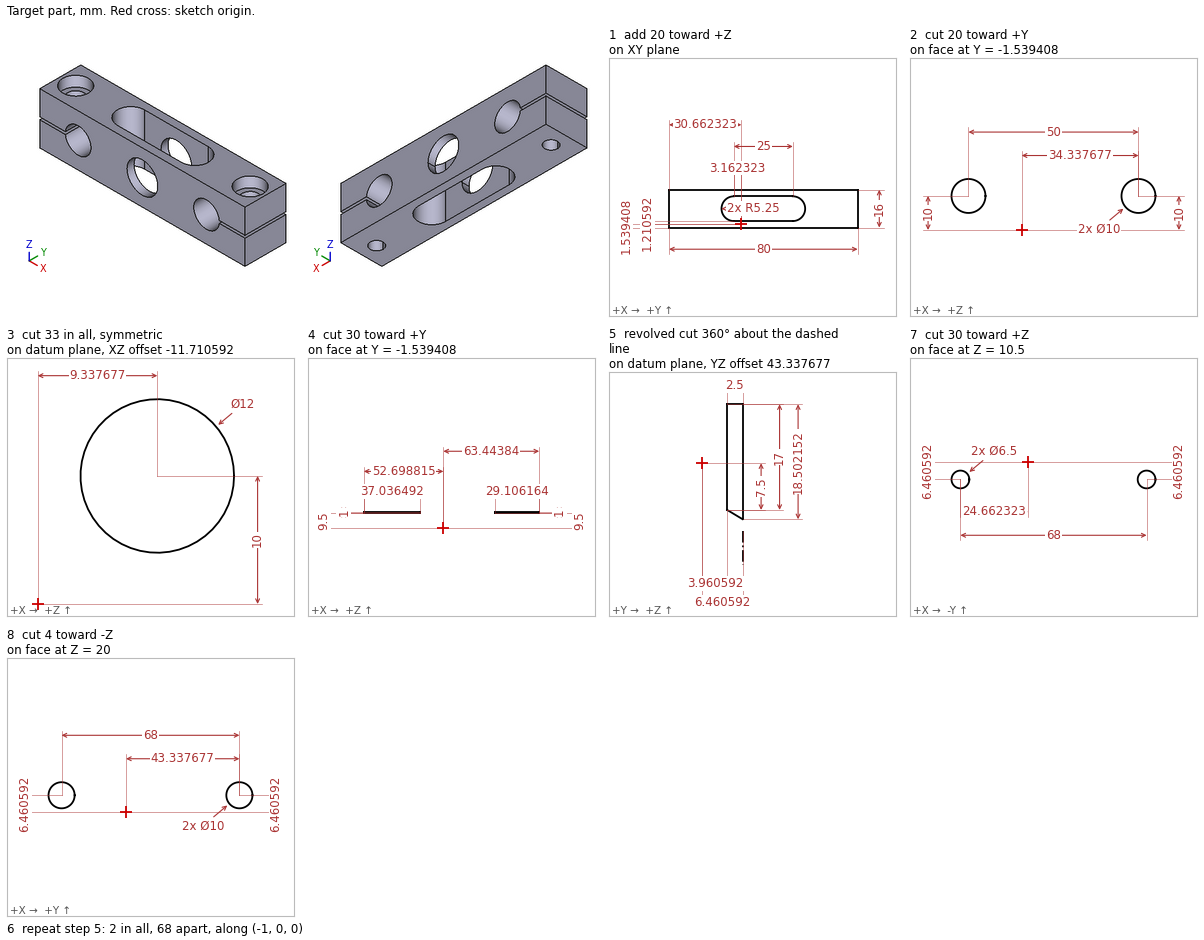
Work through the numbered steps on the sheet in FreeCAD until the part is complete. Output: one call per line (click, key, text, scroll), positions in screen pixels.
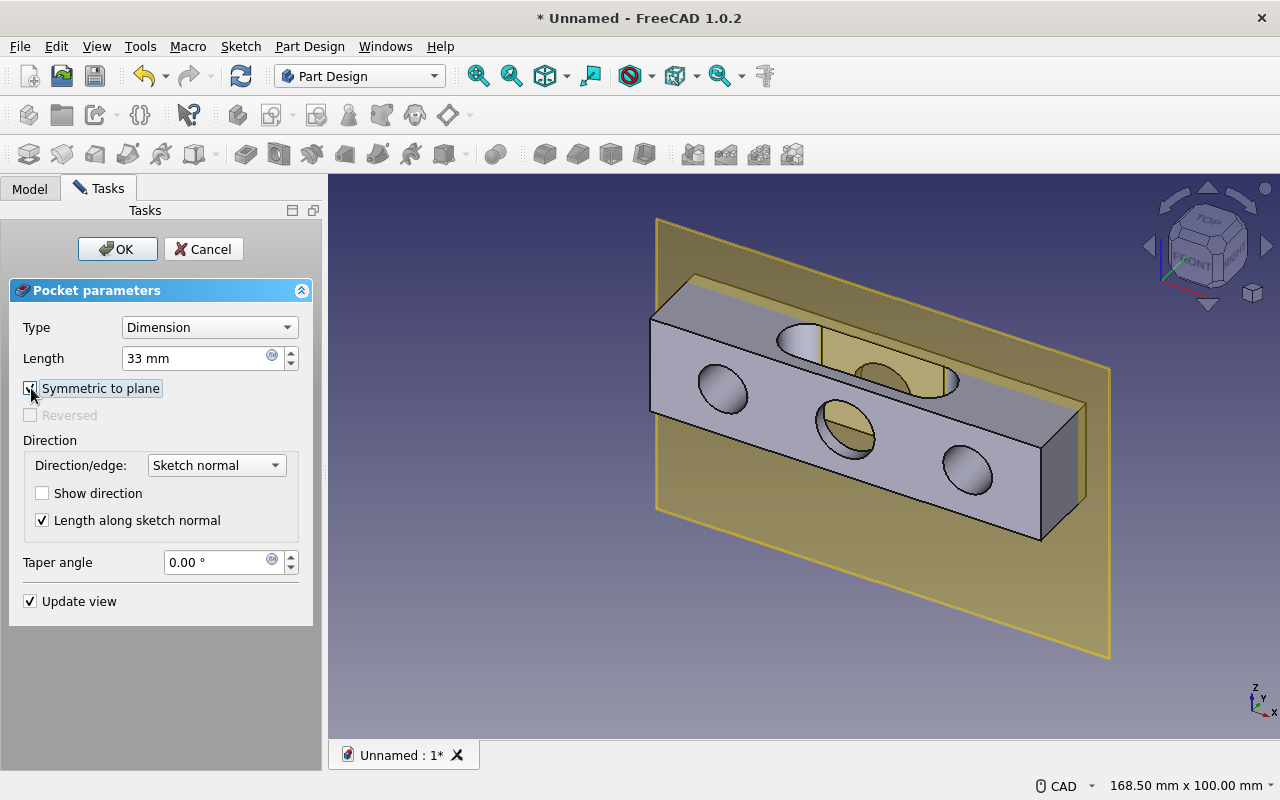
click(118, 249)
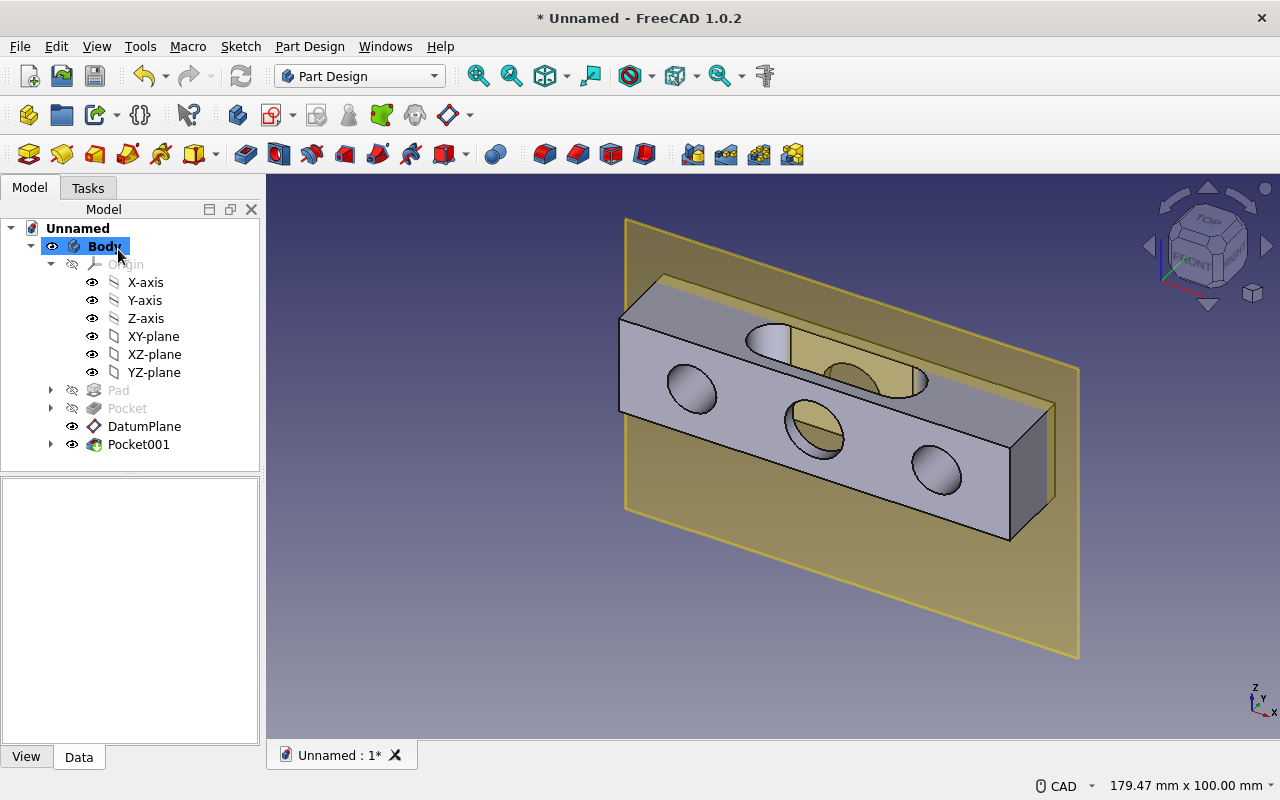
click(117, 426)
key(space)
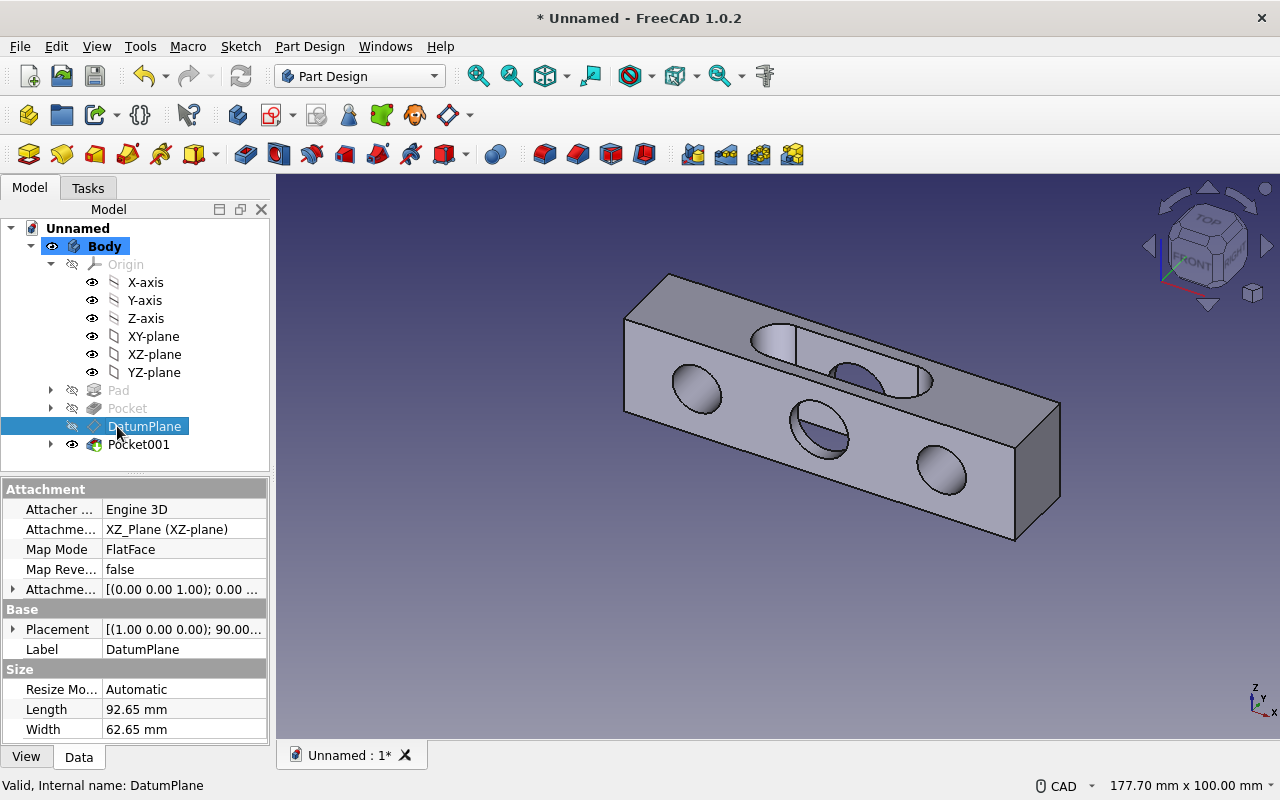
click(875, 460)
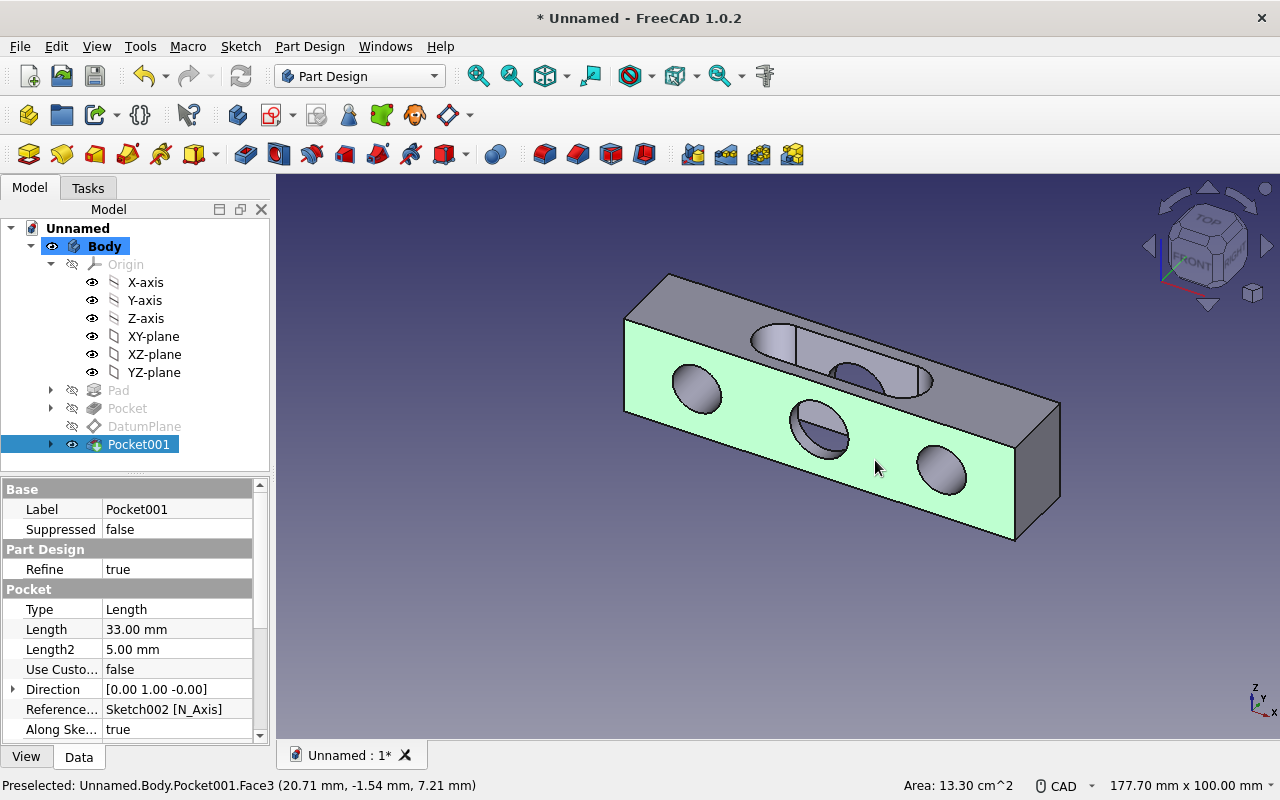
click(270, 116)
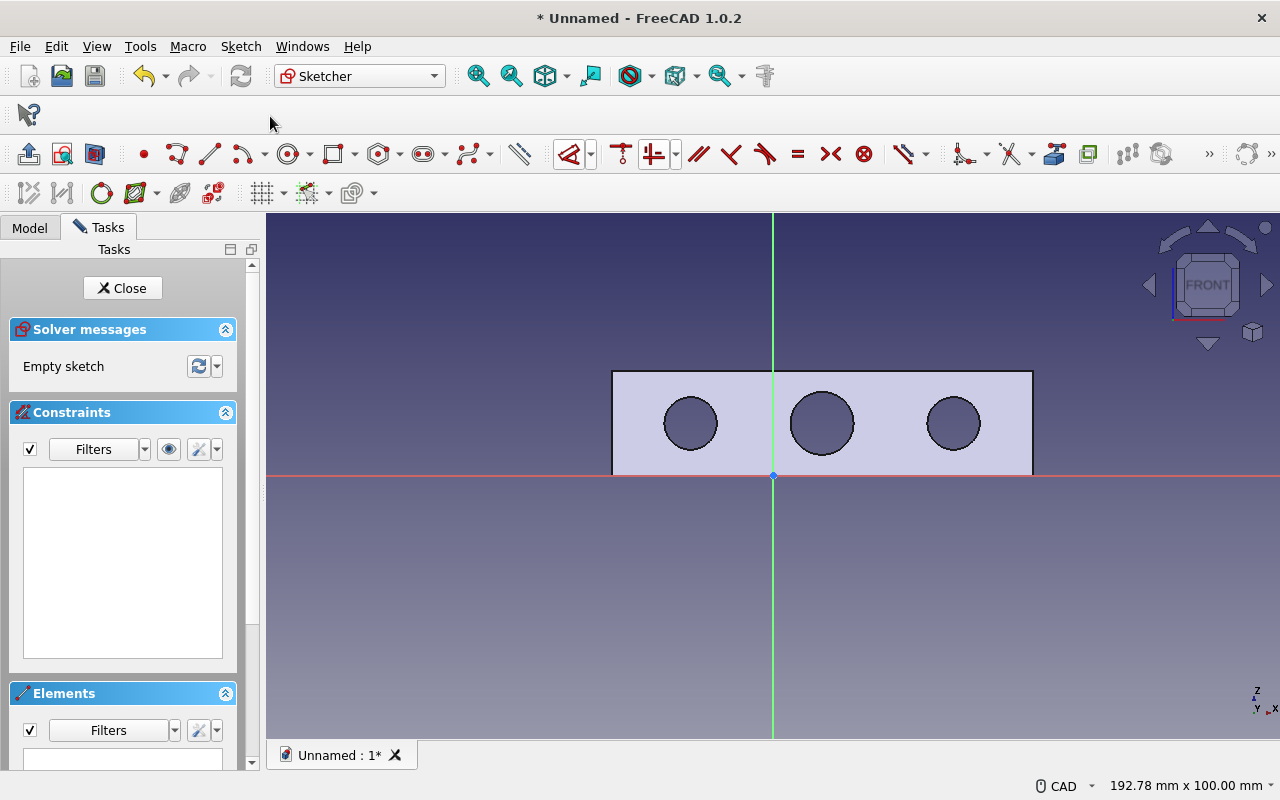
scroll(294, 601, down, 1)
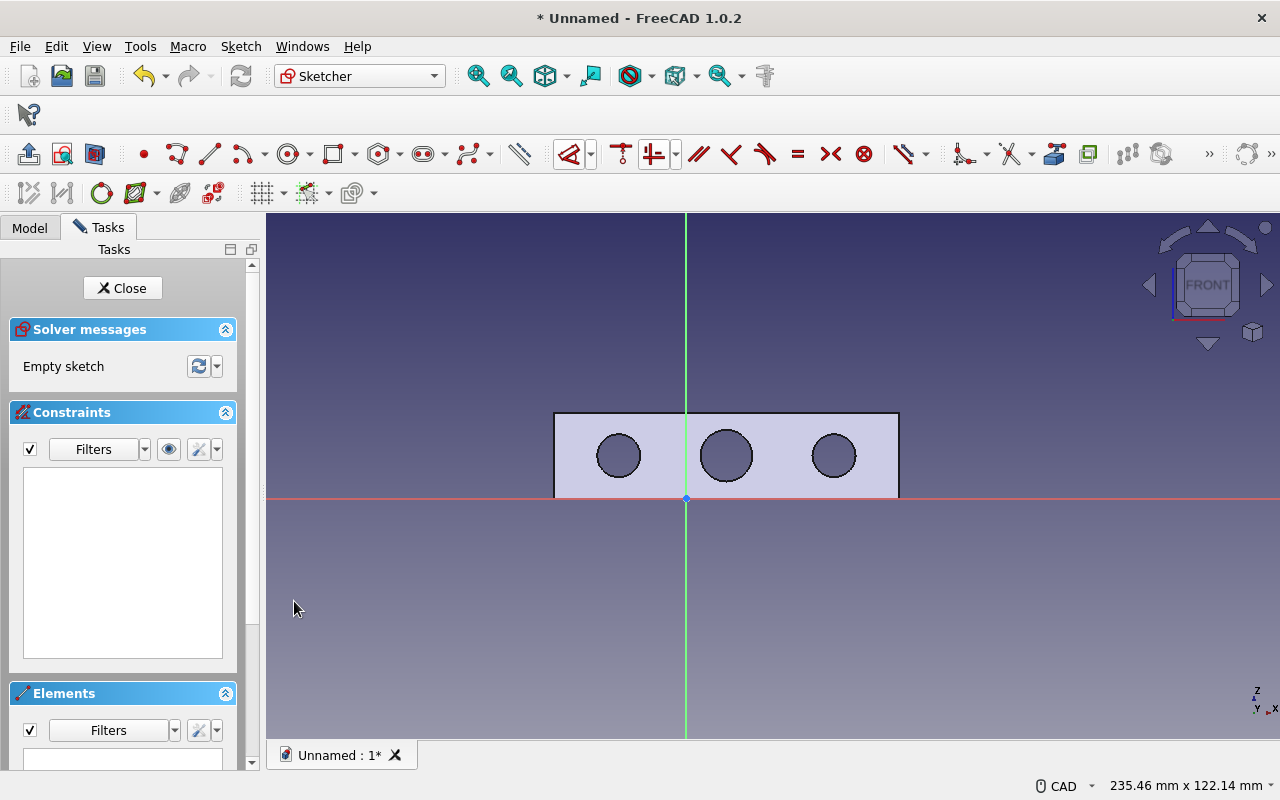
key(g)
key(r)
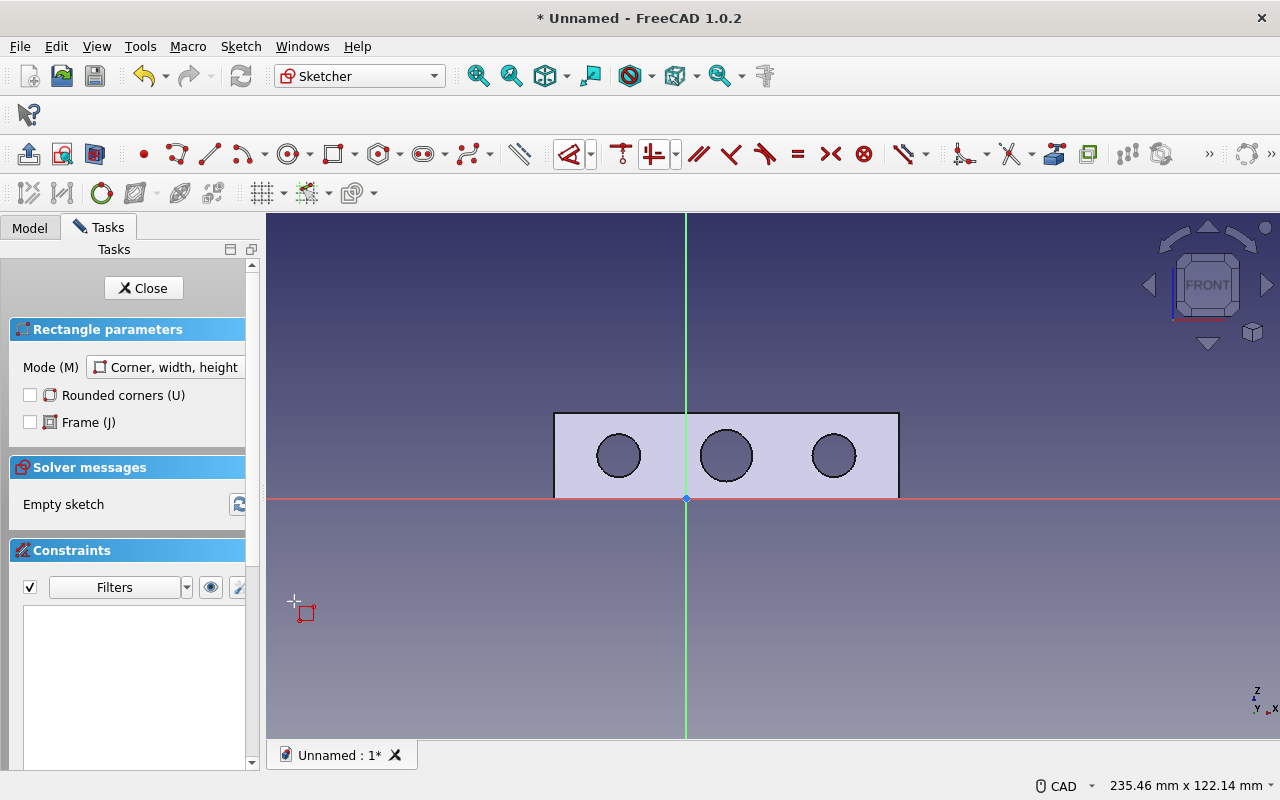
scroll(834, 454, up, 7)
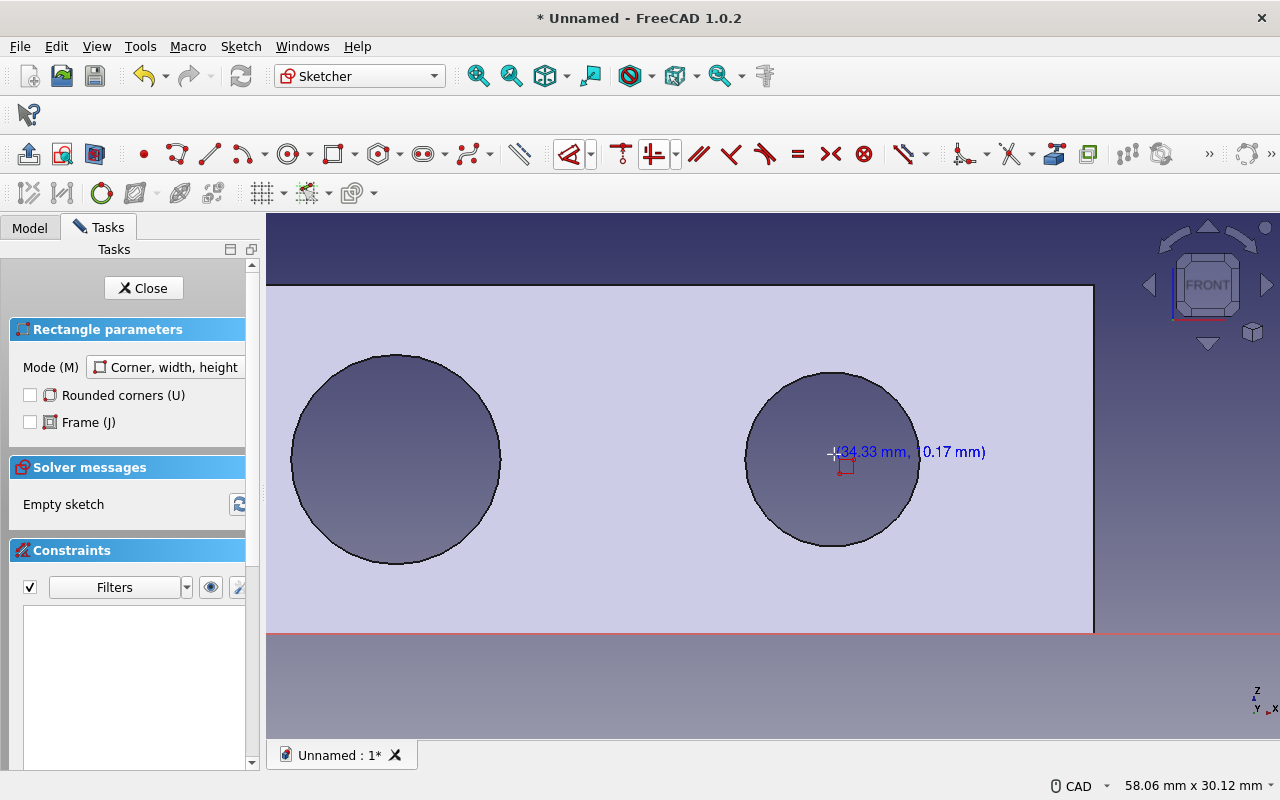
scroll(867, 447, down, 6)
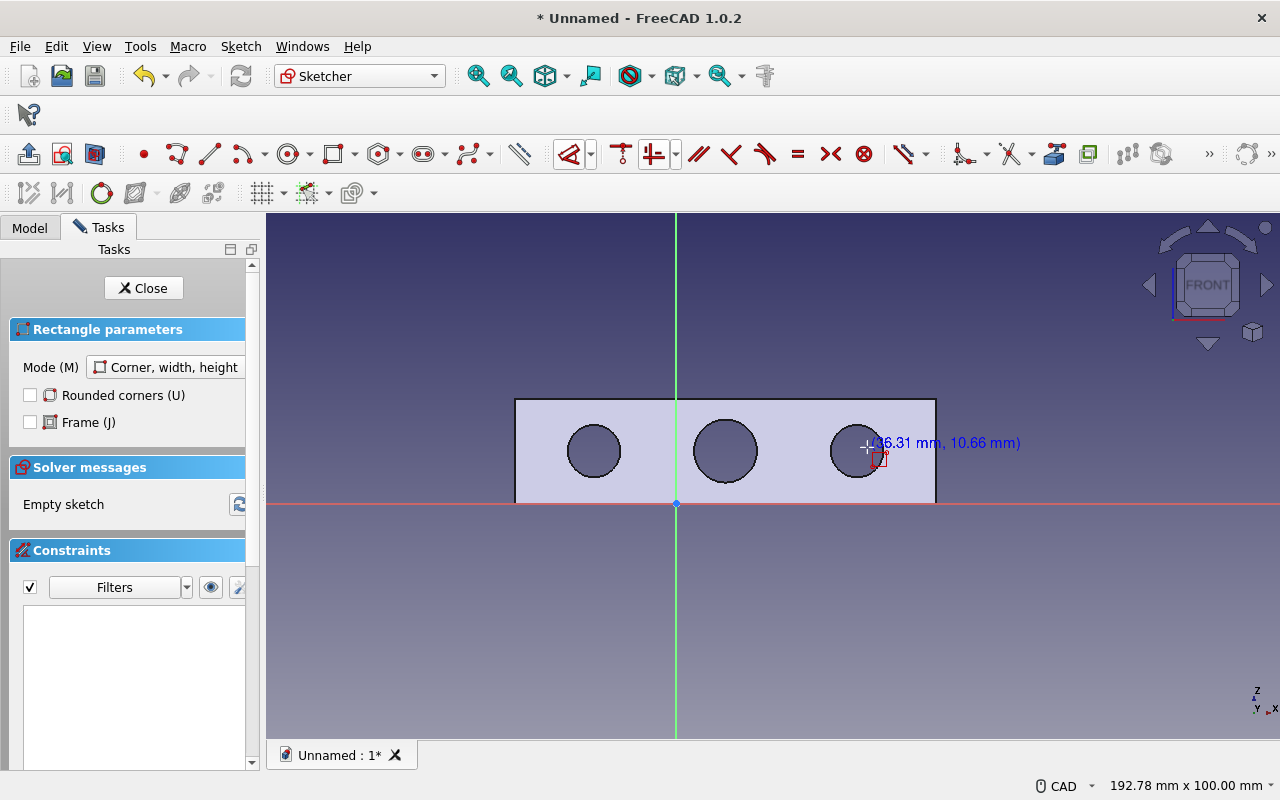
click(857, 448)
move(1010, 454)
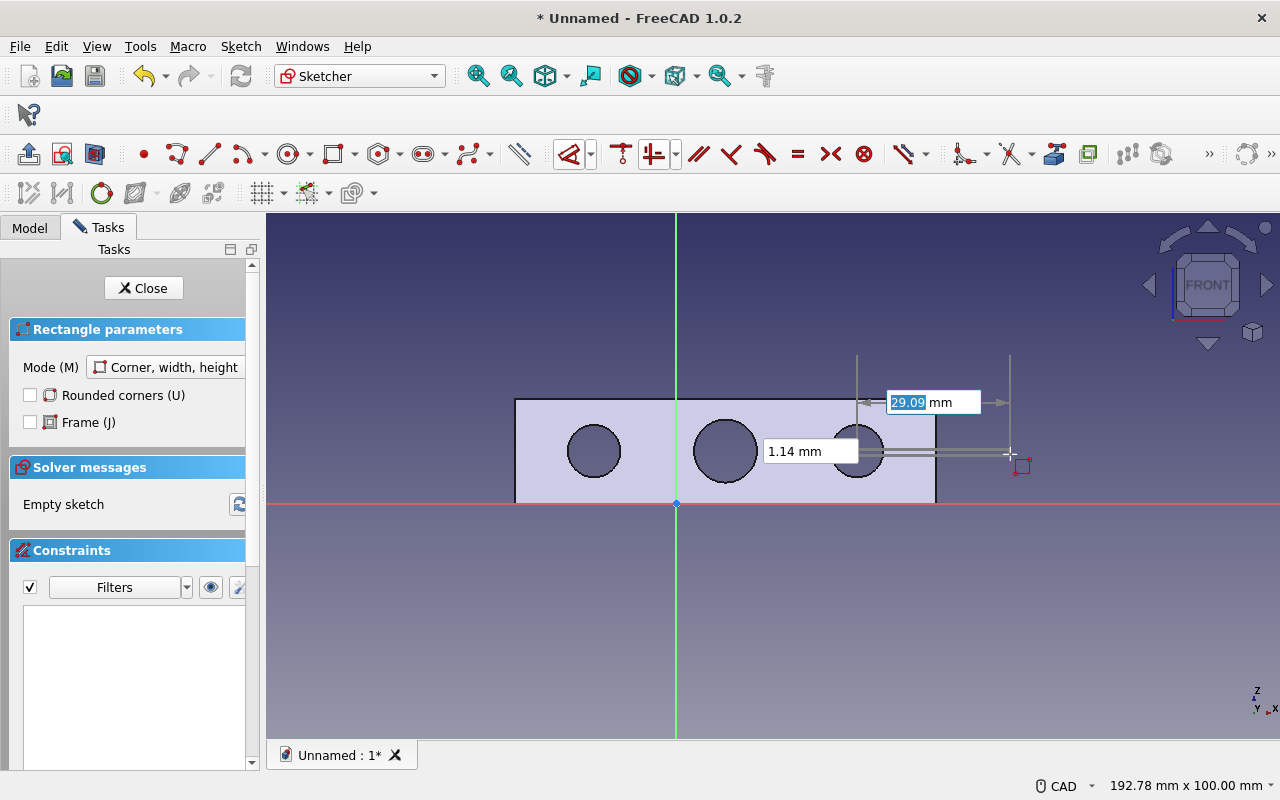
text(29.106164)
key(Tab)
text(1)
key(Return)